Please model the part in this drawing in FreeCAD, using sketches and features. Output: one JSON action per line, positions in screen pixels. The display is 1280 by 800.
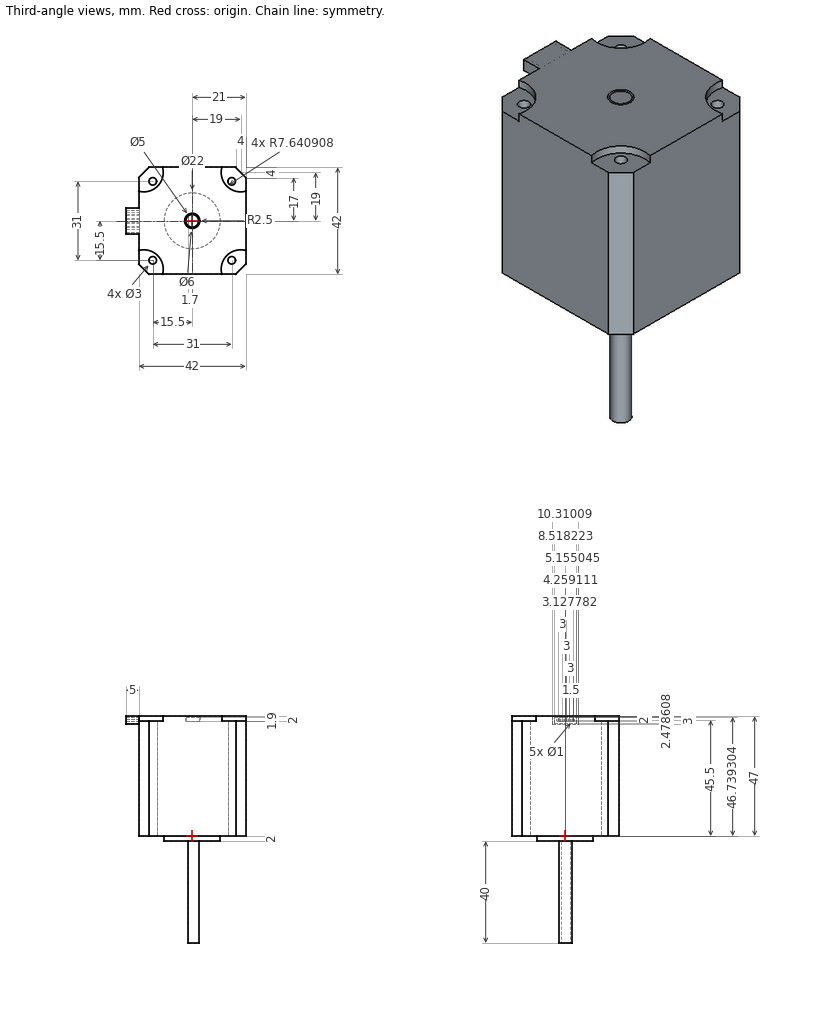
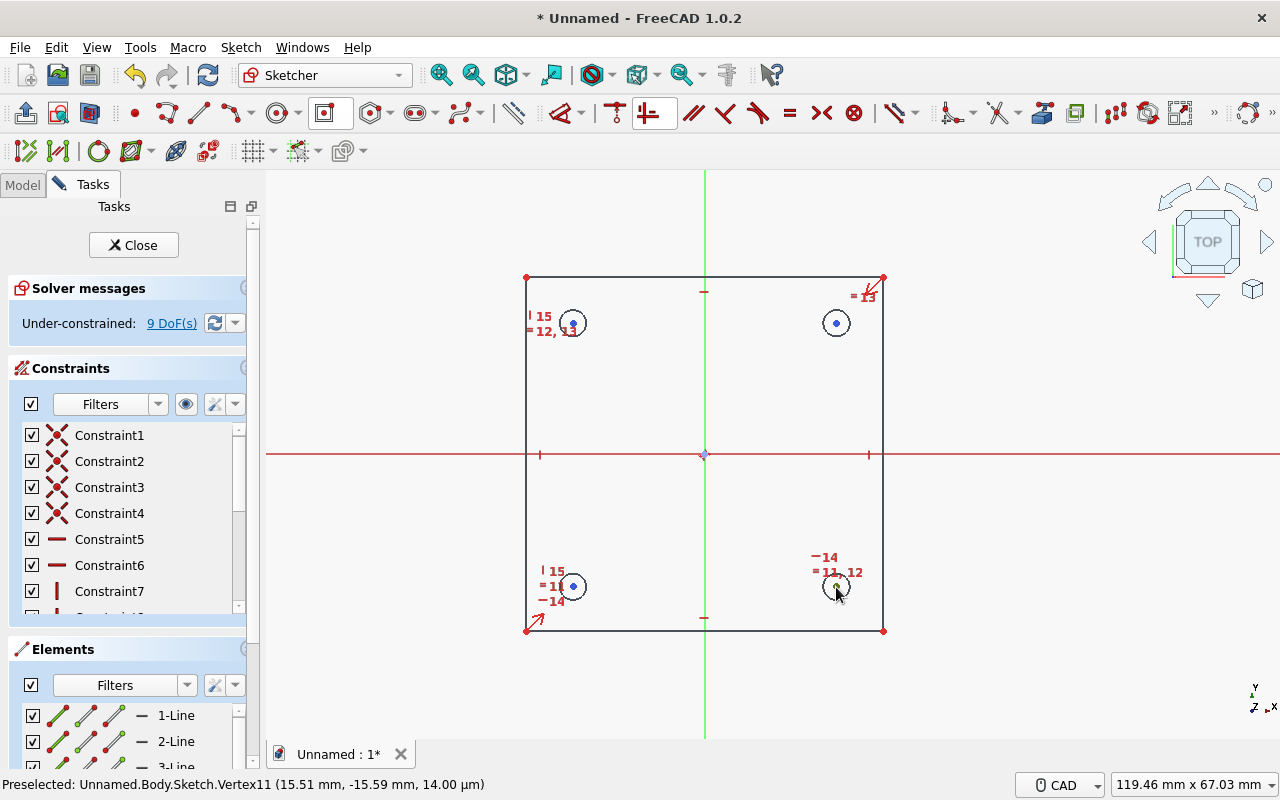
{"action": "left_click", "coordinate": [837, 323]}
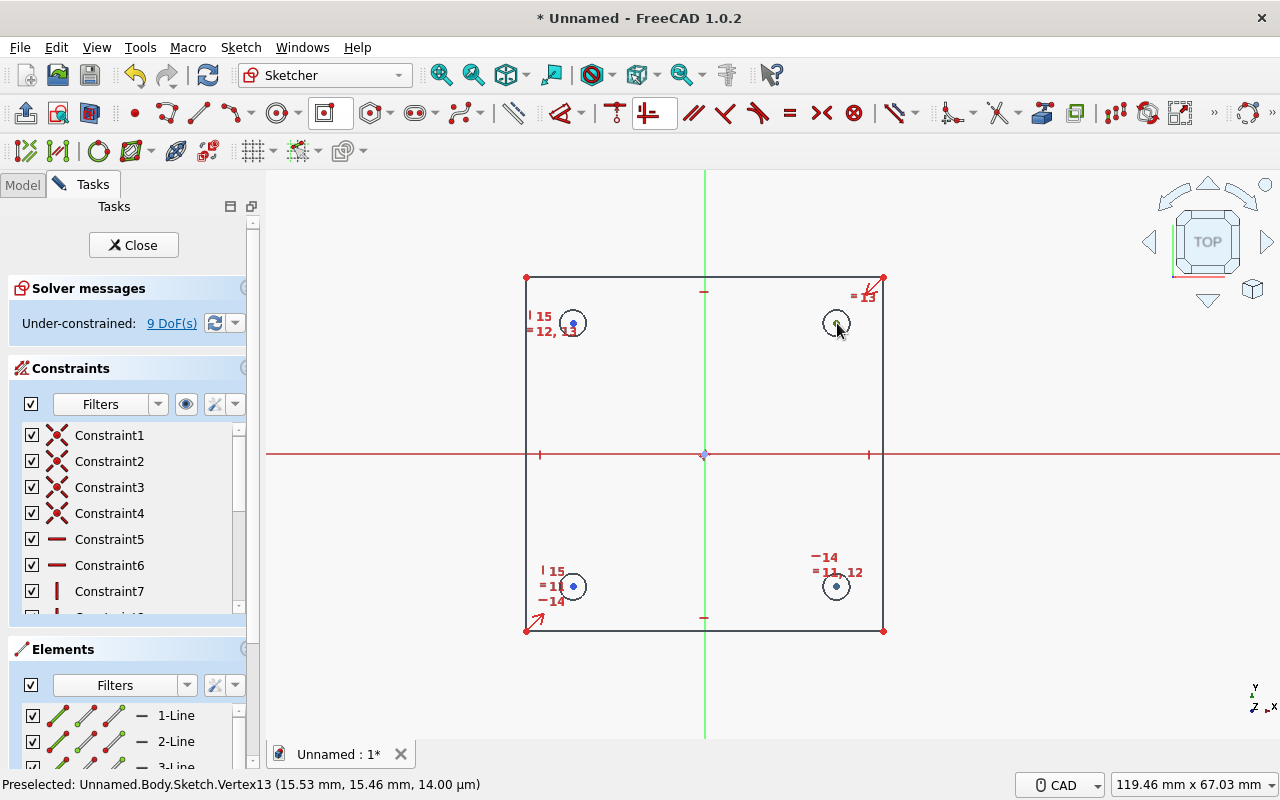
{"action": "key", "text": "v"}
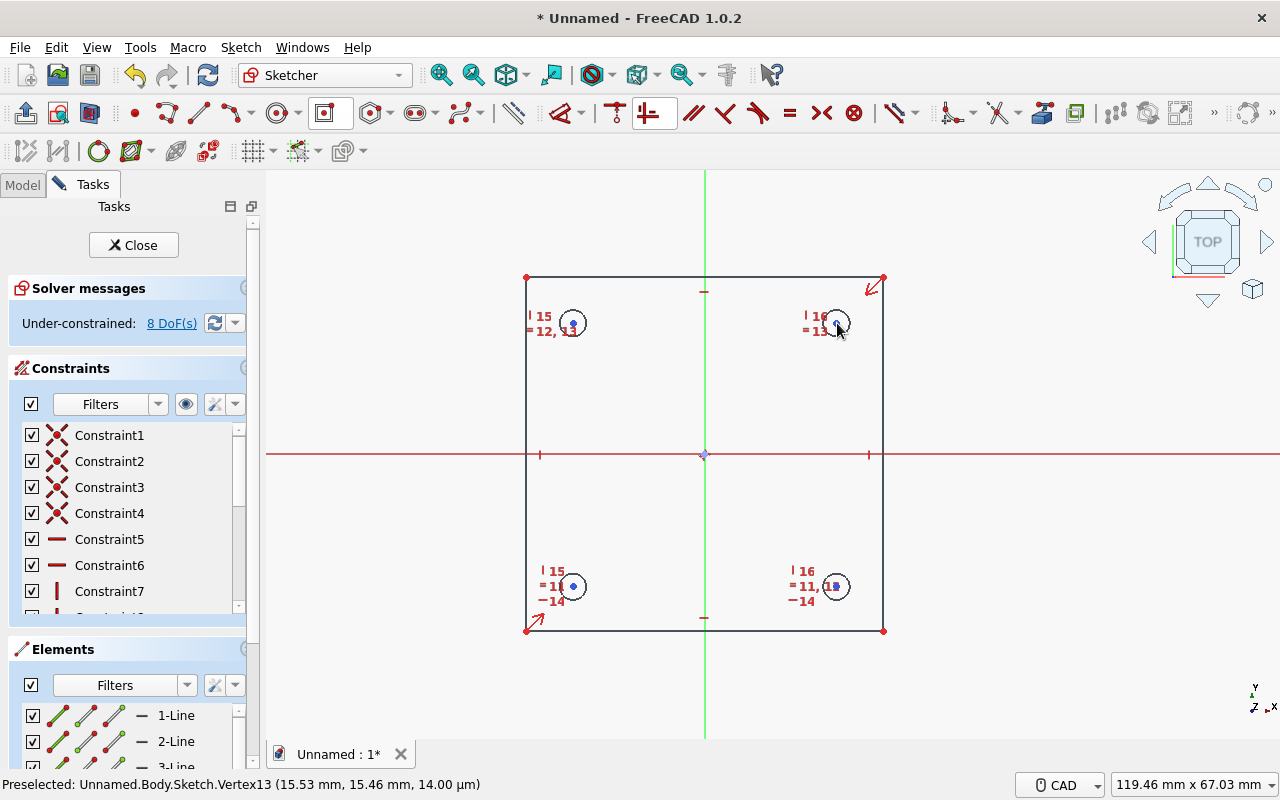
{"action": "scroll", "coordinate": [573, 323], "scroll_direction": "up", "scroll_amount": 4}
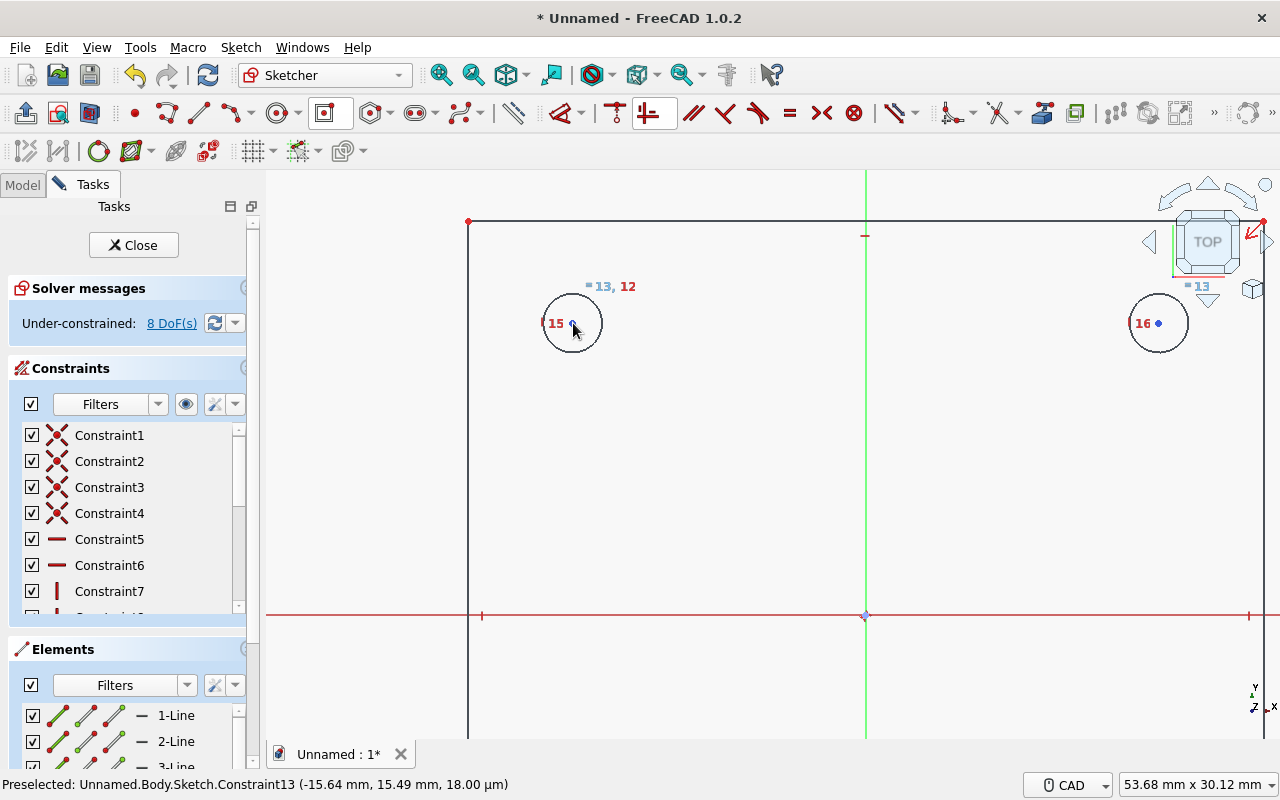
{"action": "left_click", "coordinate": [573, 323]}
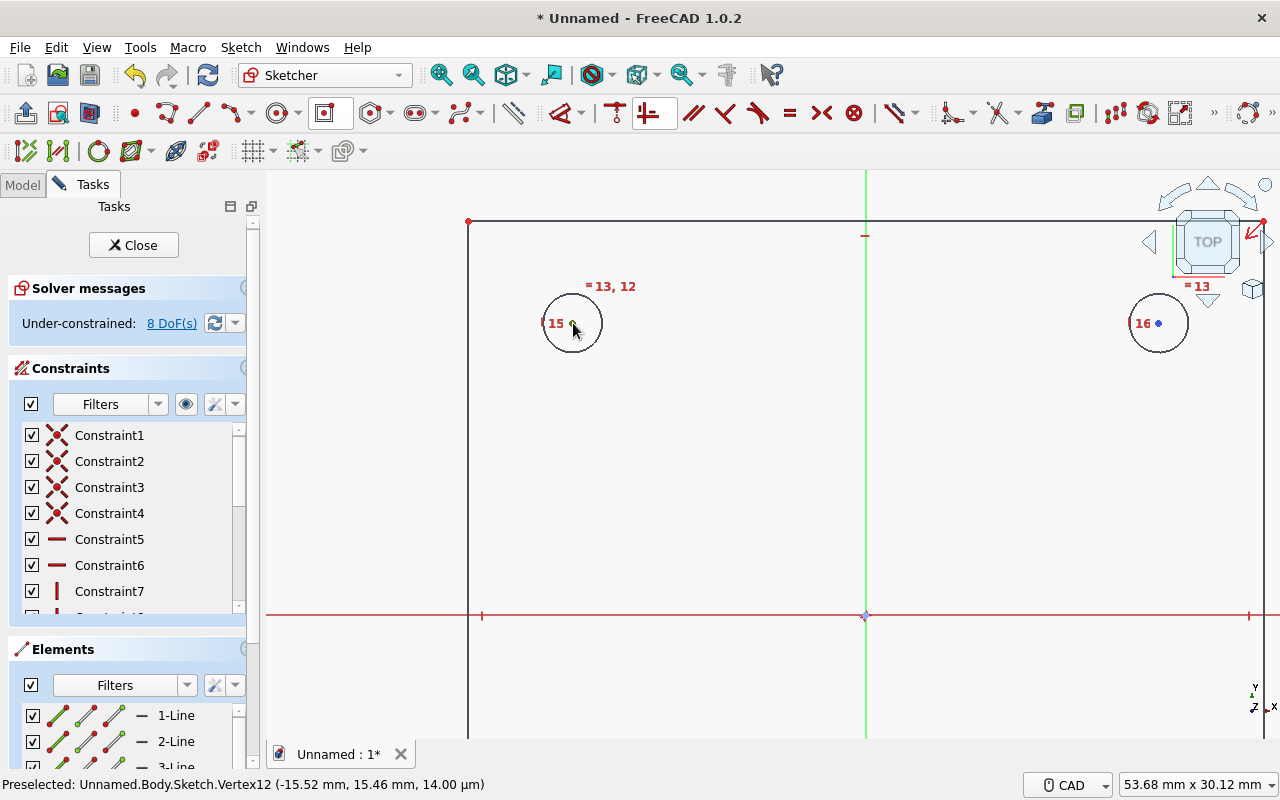
{"action": "scroll", "coordinate": [573, 323], "scroll_direction": "down", "scroll_amount": 4}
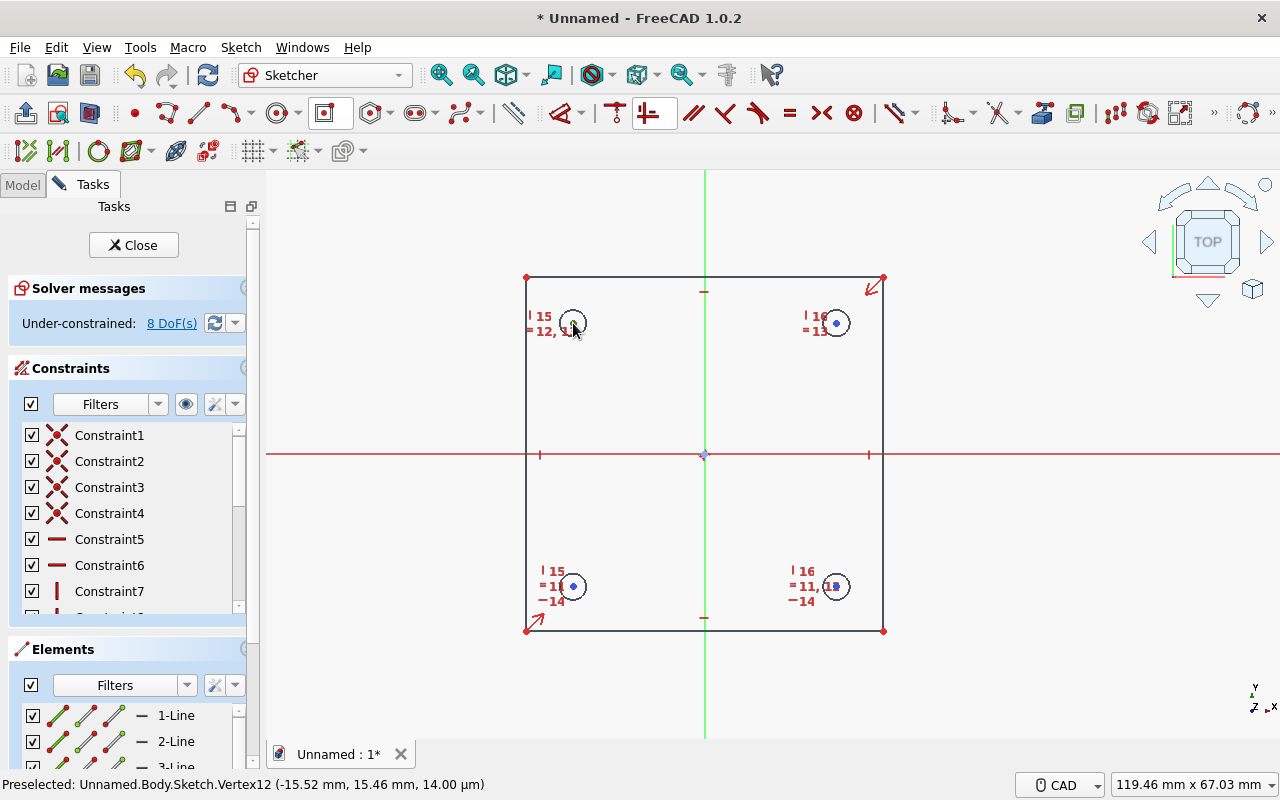
{"action": "left_click", "coordinate": [836, 323]}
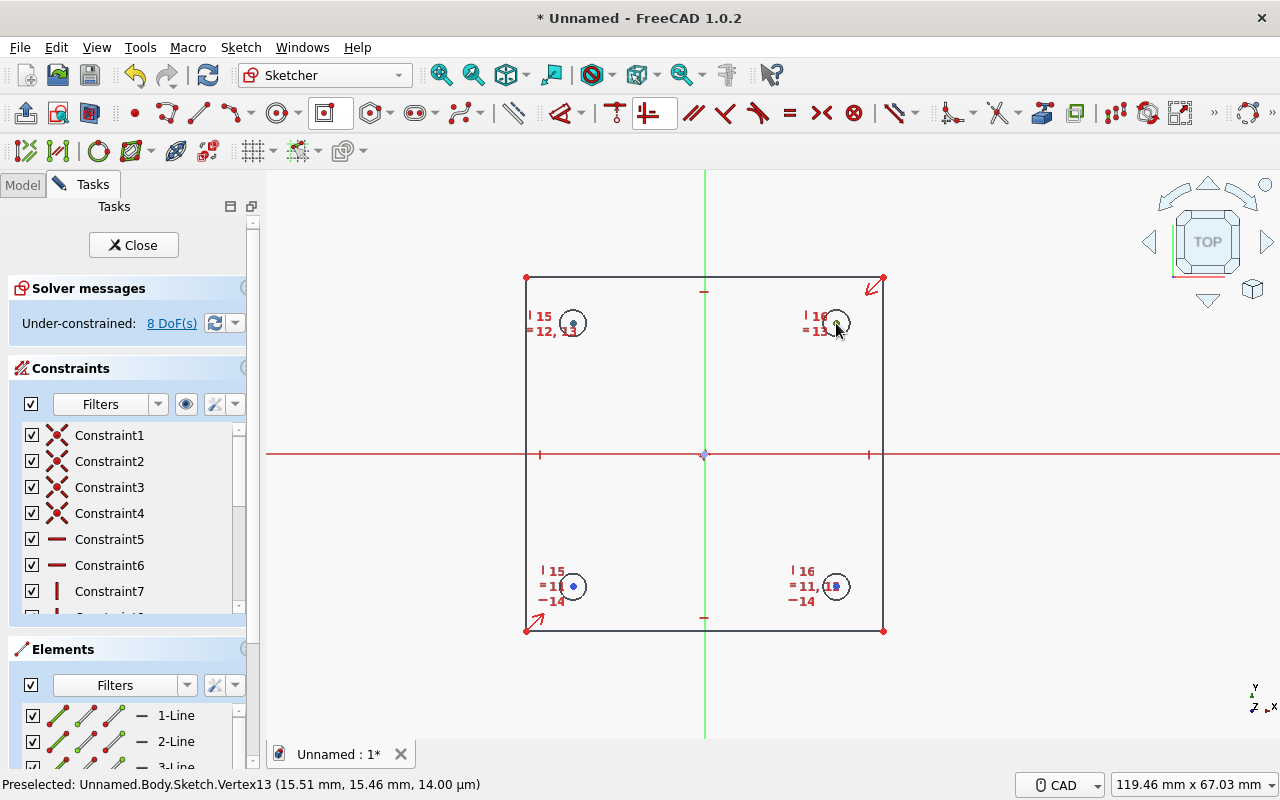
{"action": "key", "text": "h"}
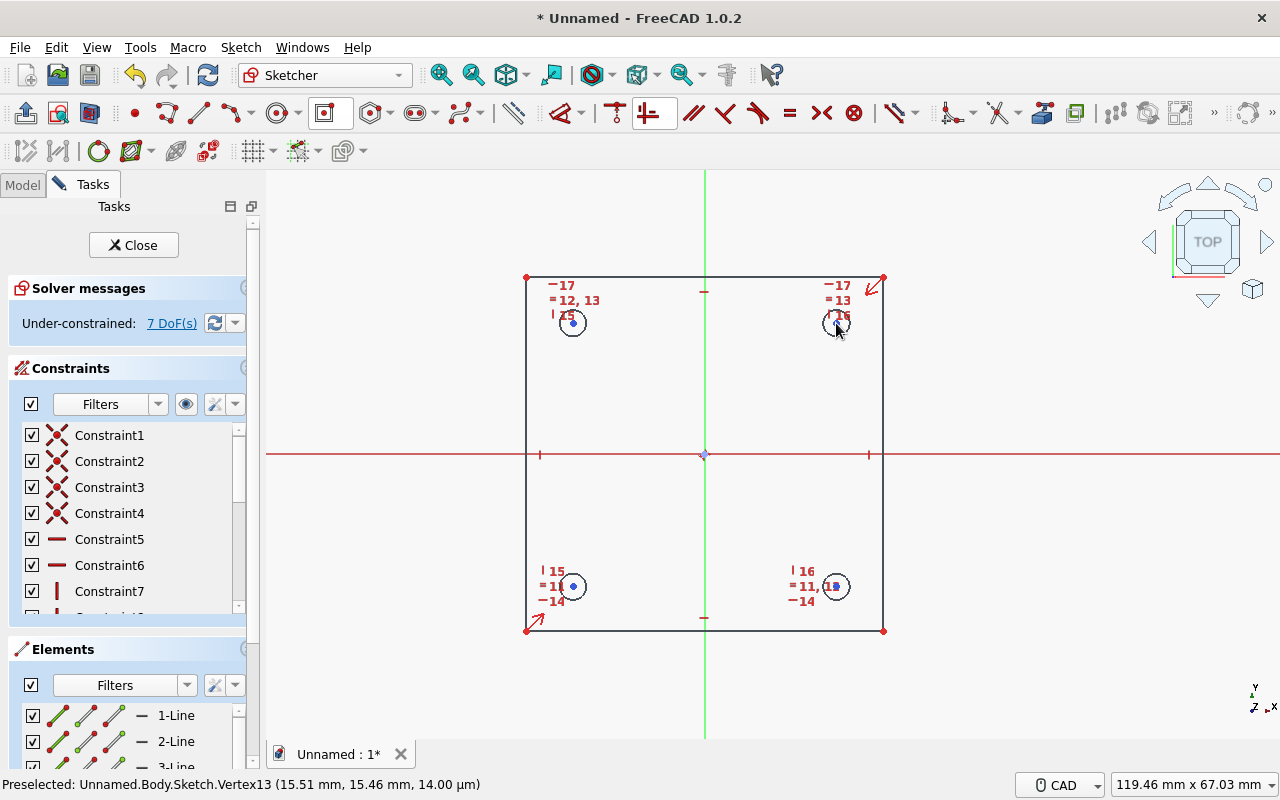
{"action": "left_click", "coordinate": [560, 114]}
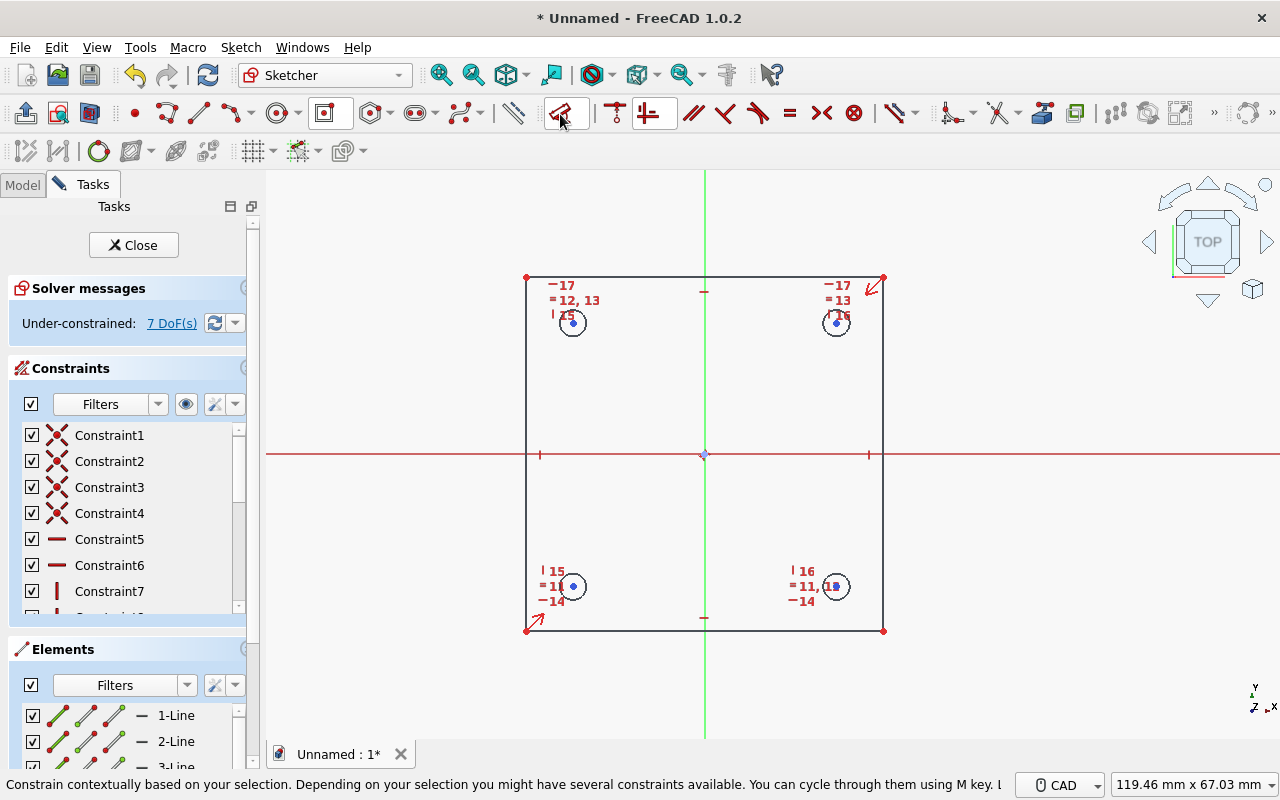
{"action": "scroll", "coordinate": [582, 577], "scroll_direction": "up", "scroll_amount": 3}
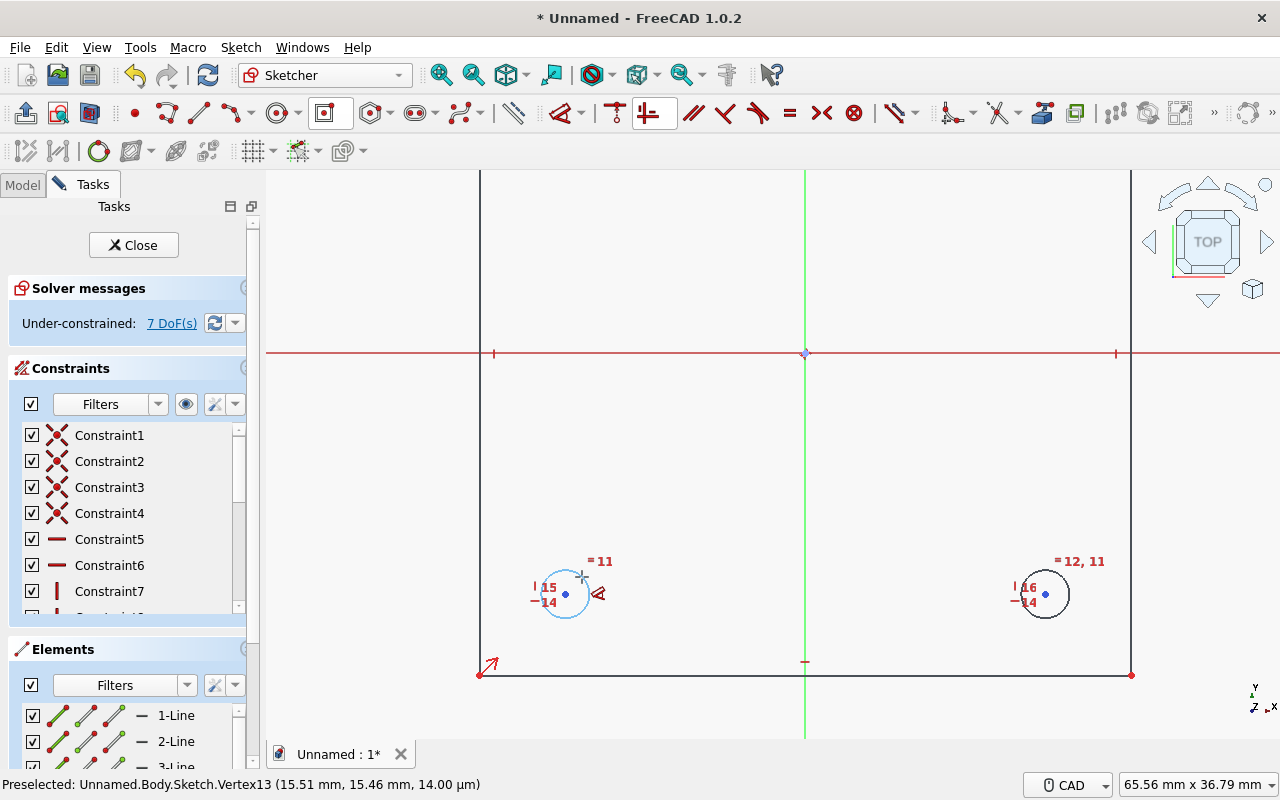
{"action": "left_click", "coordinate": [582, 577]}
{"action": "left_click", "coordinate": [604, 554]}